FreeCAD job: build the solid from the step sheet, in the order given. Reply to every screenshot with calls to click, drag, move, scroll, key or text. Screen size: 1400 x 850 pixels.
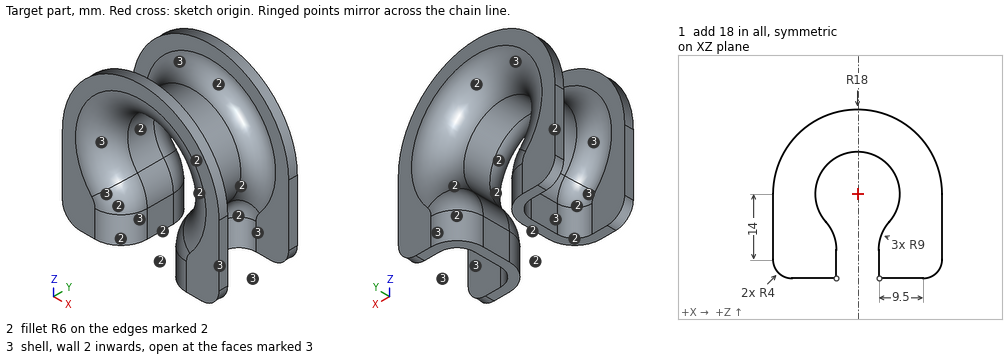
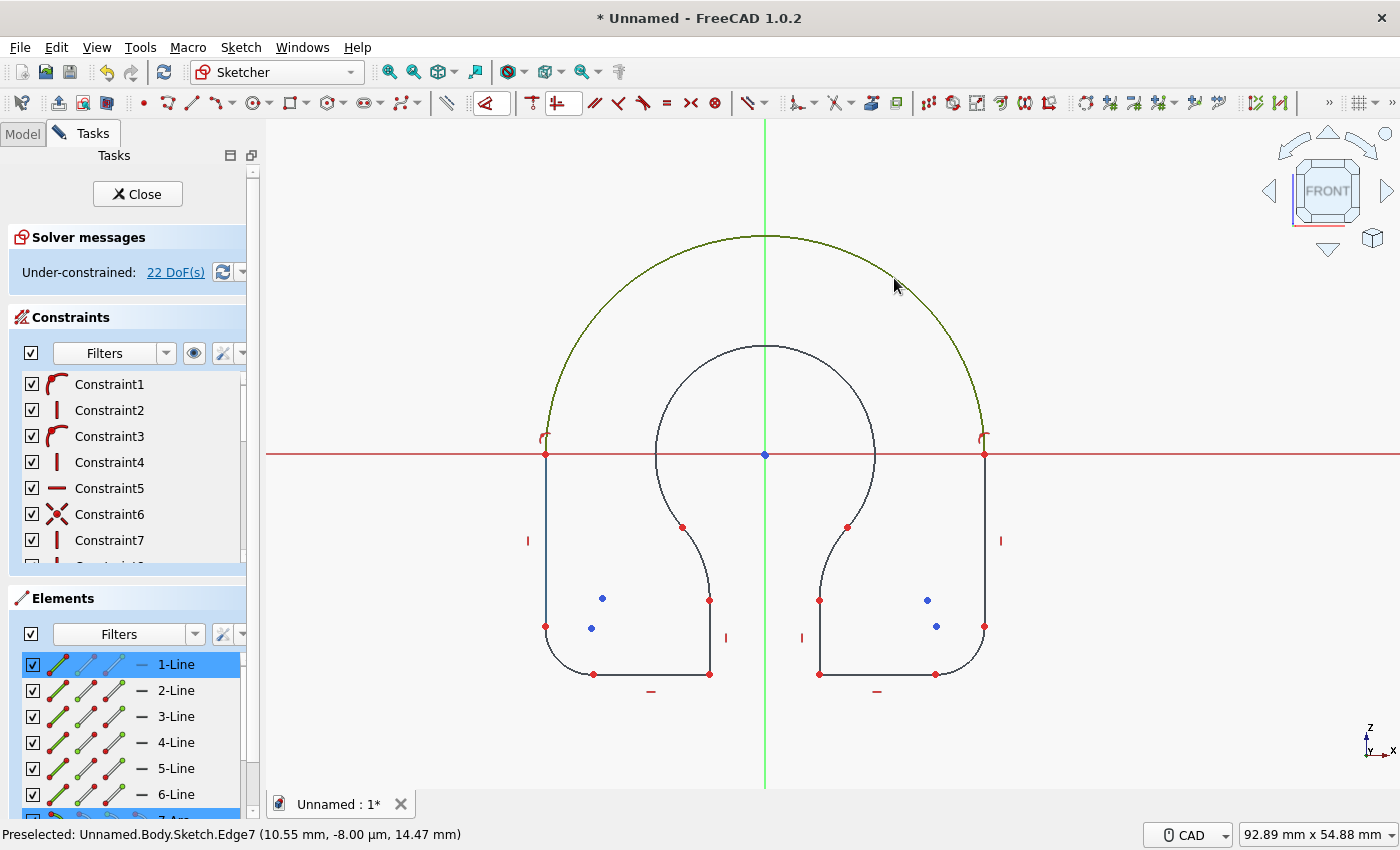
key(t)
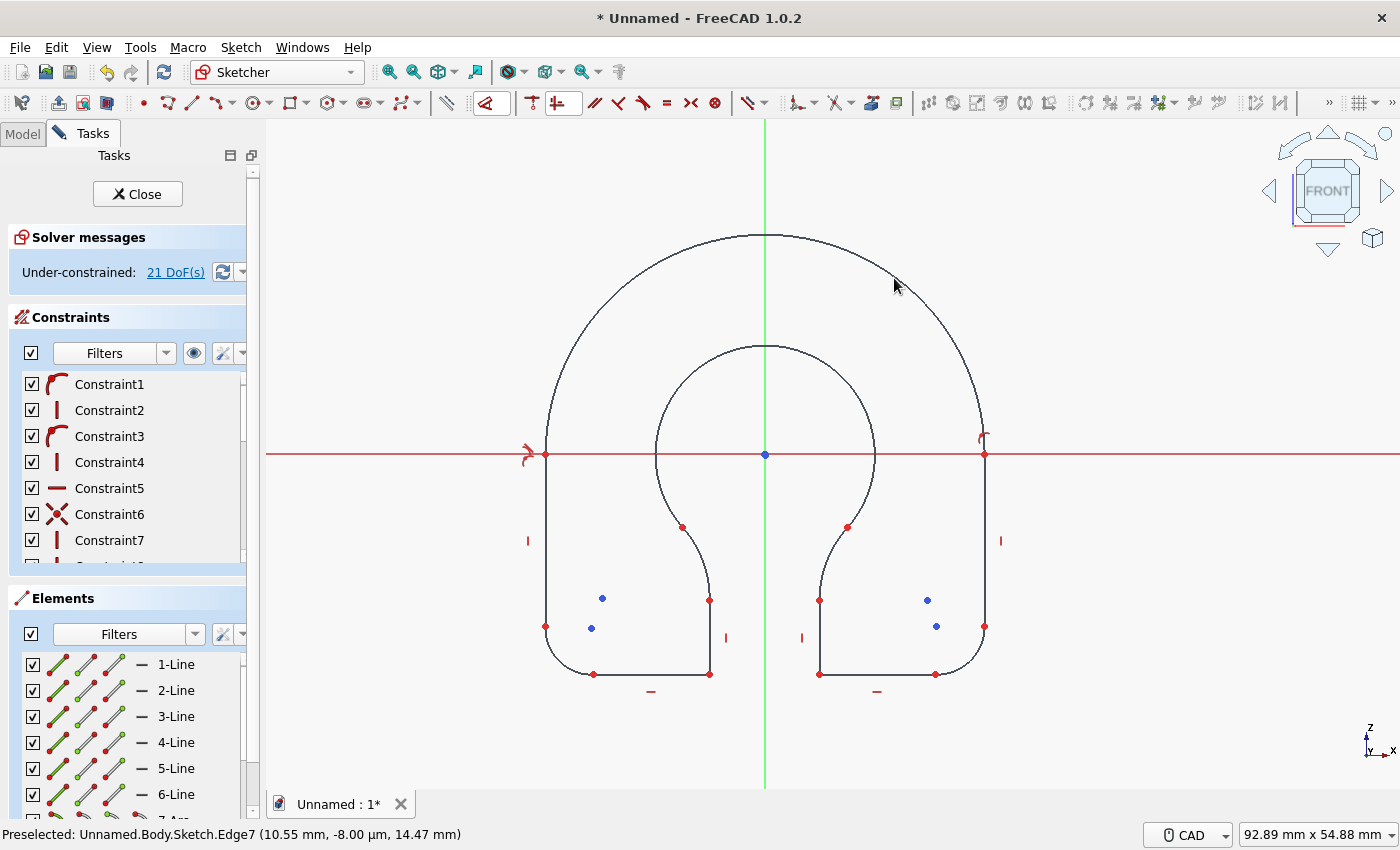
click(546, 575)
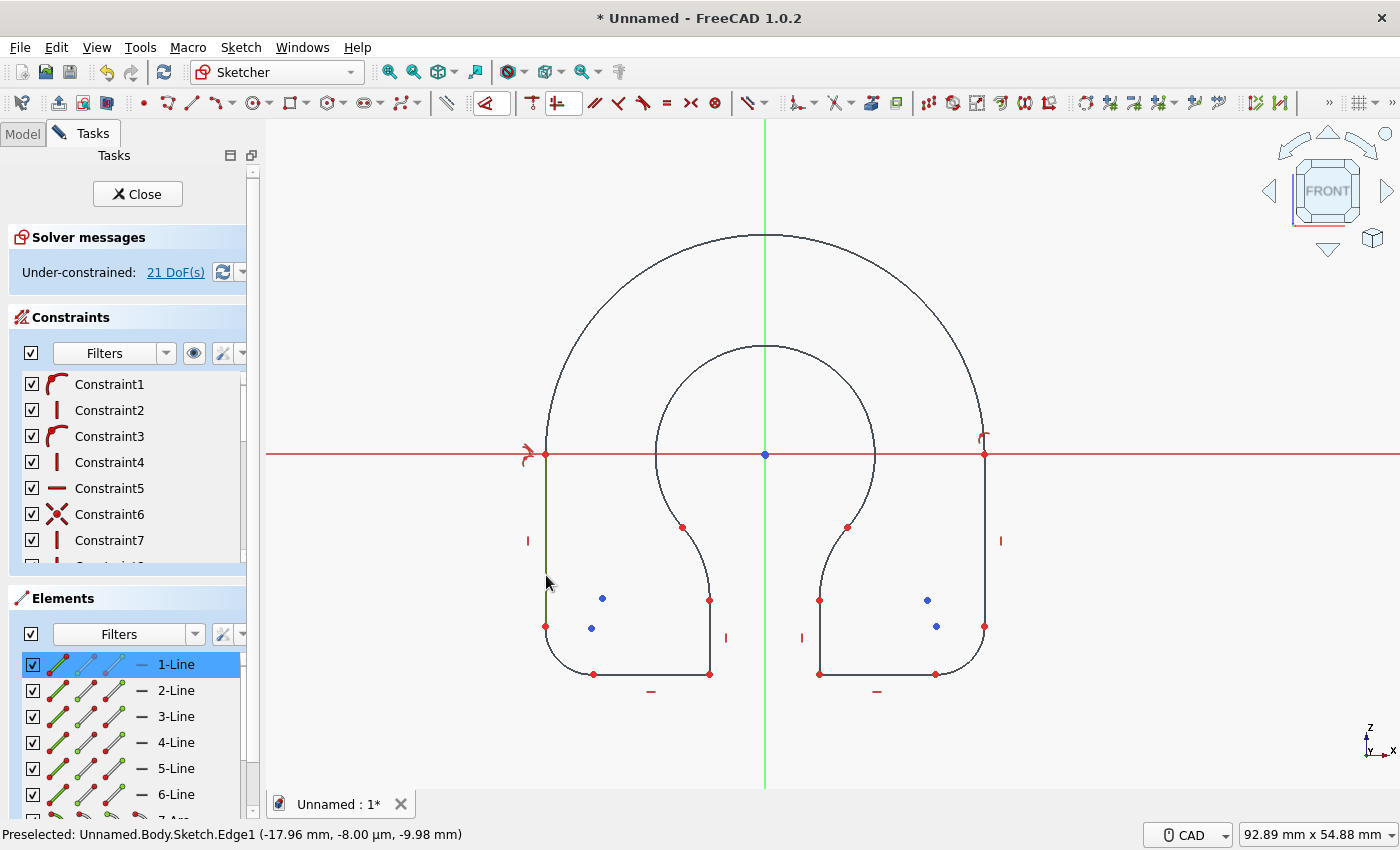
click(550, 649)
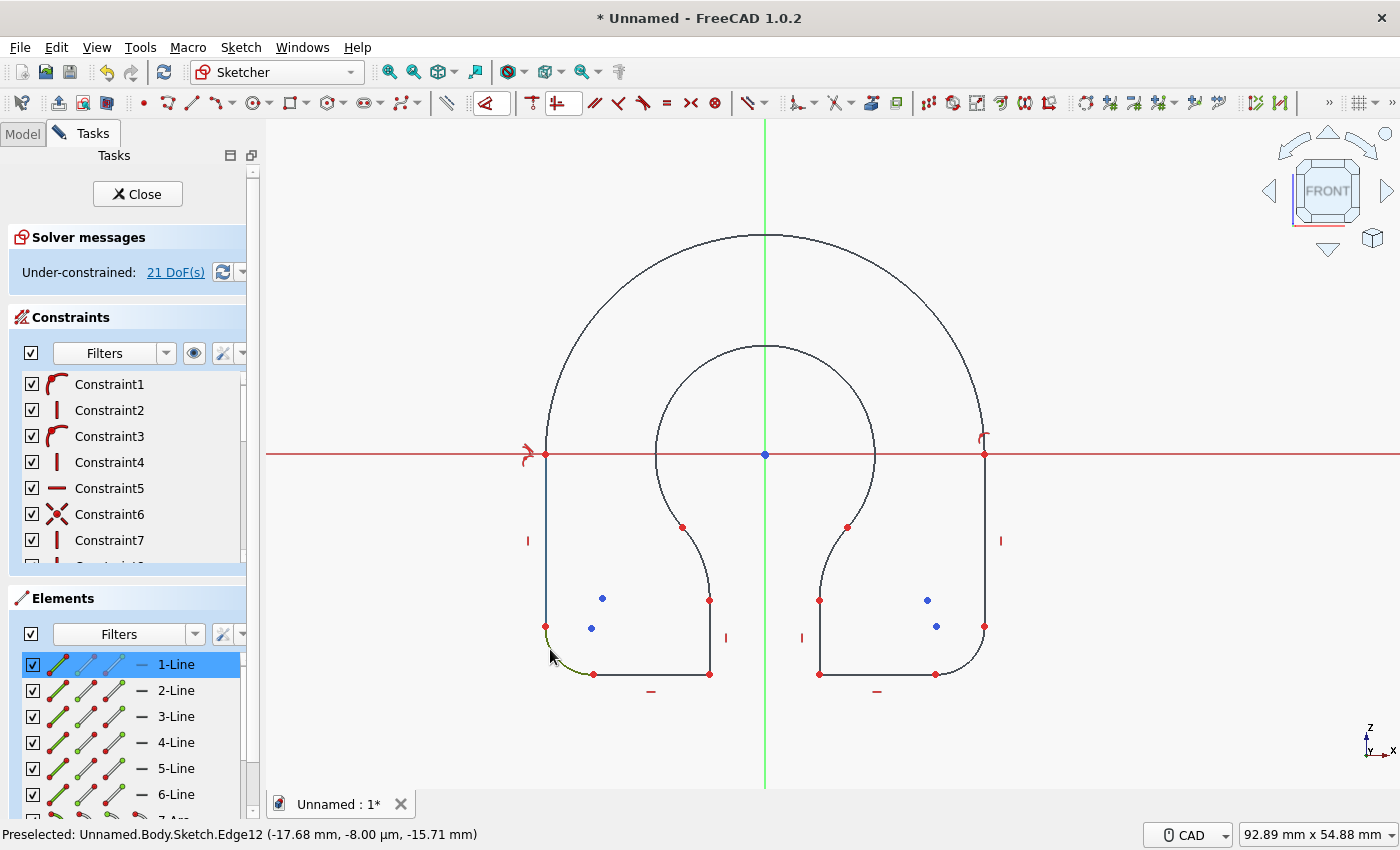
key(t)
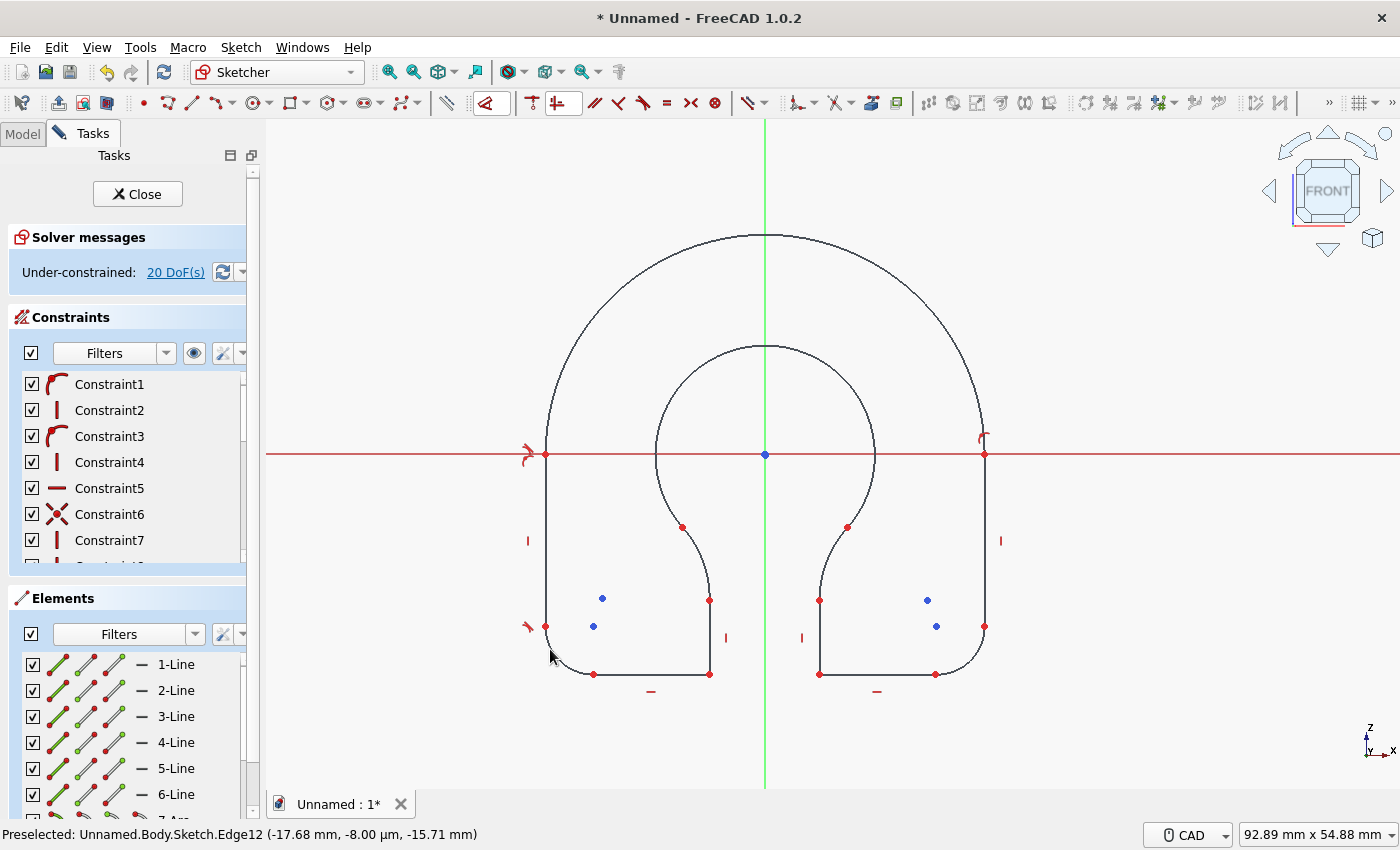
click(985, 506)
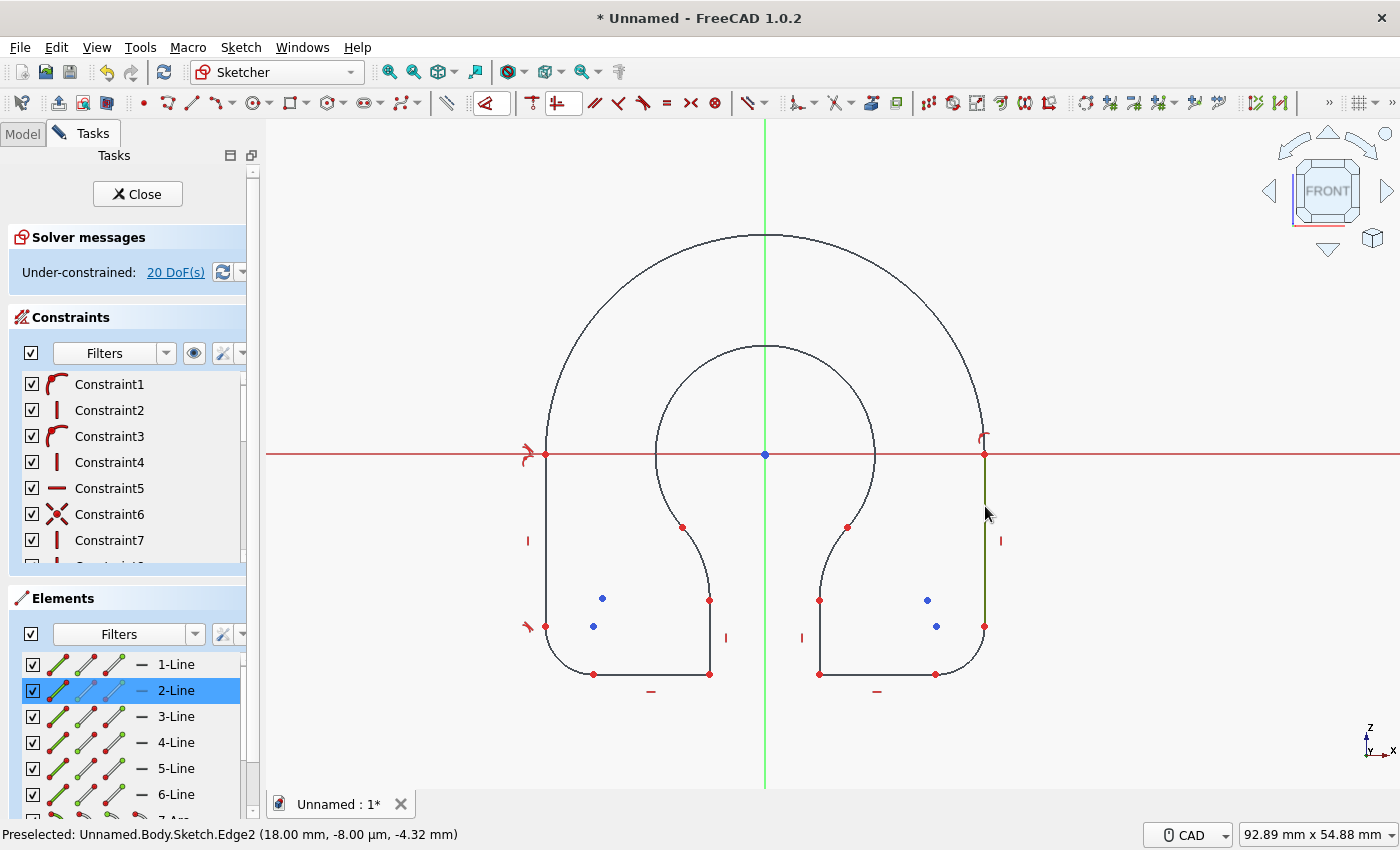
click(958, 670)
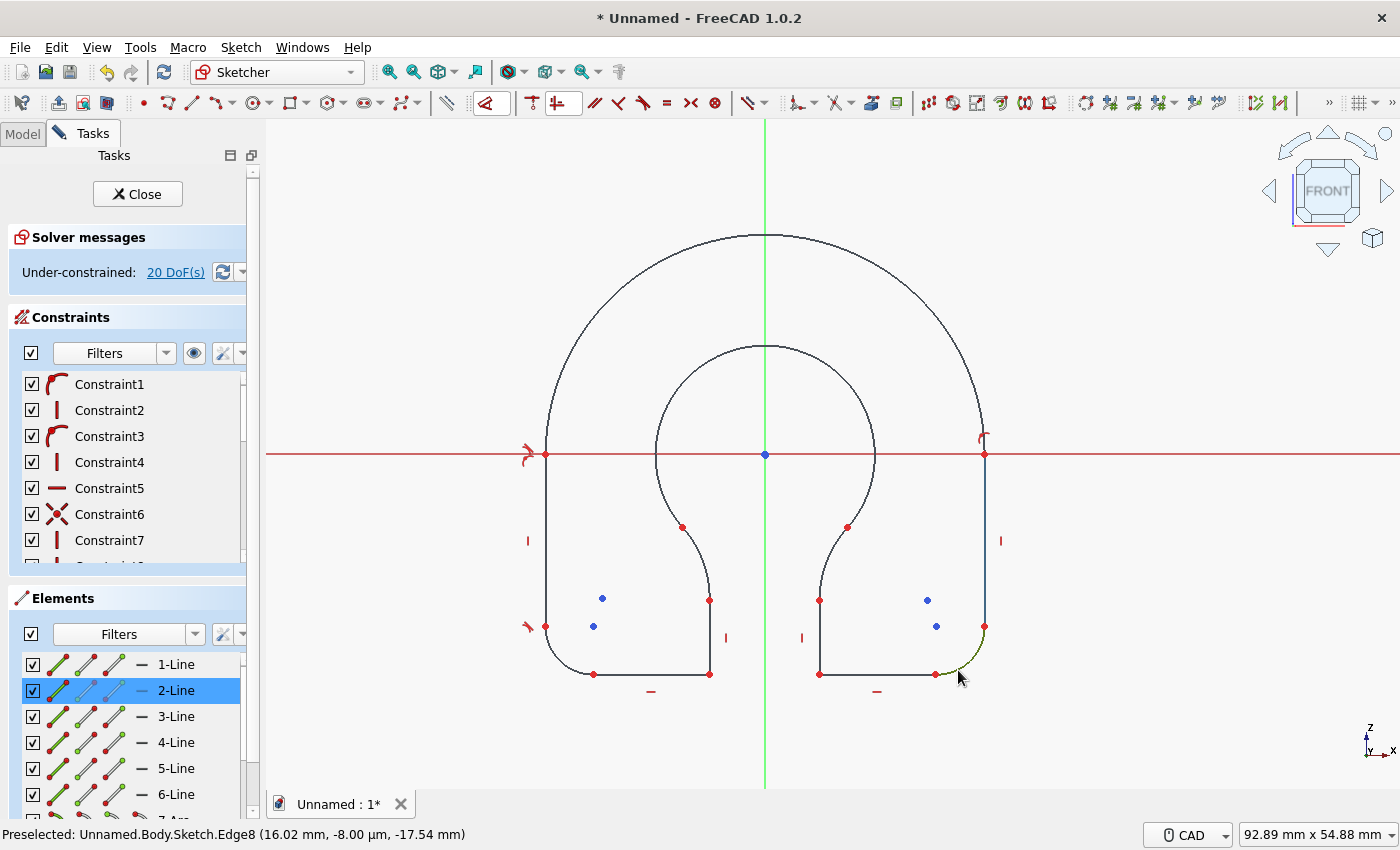
click(644, 104)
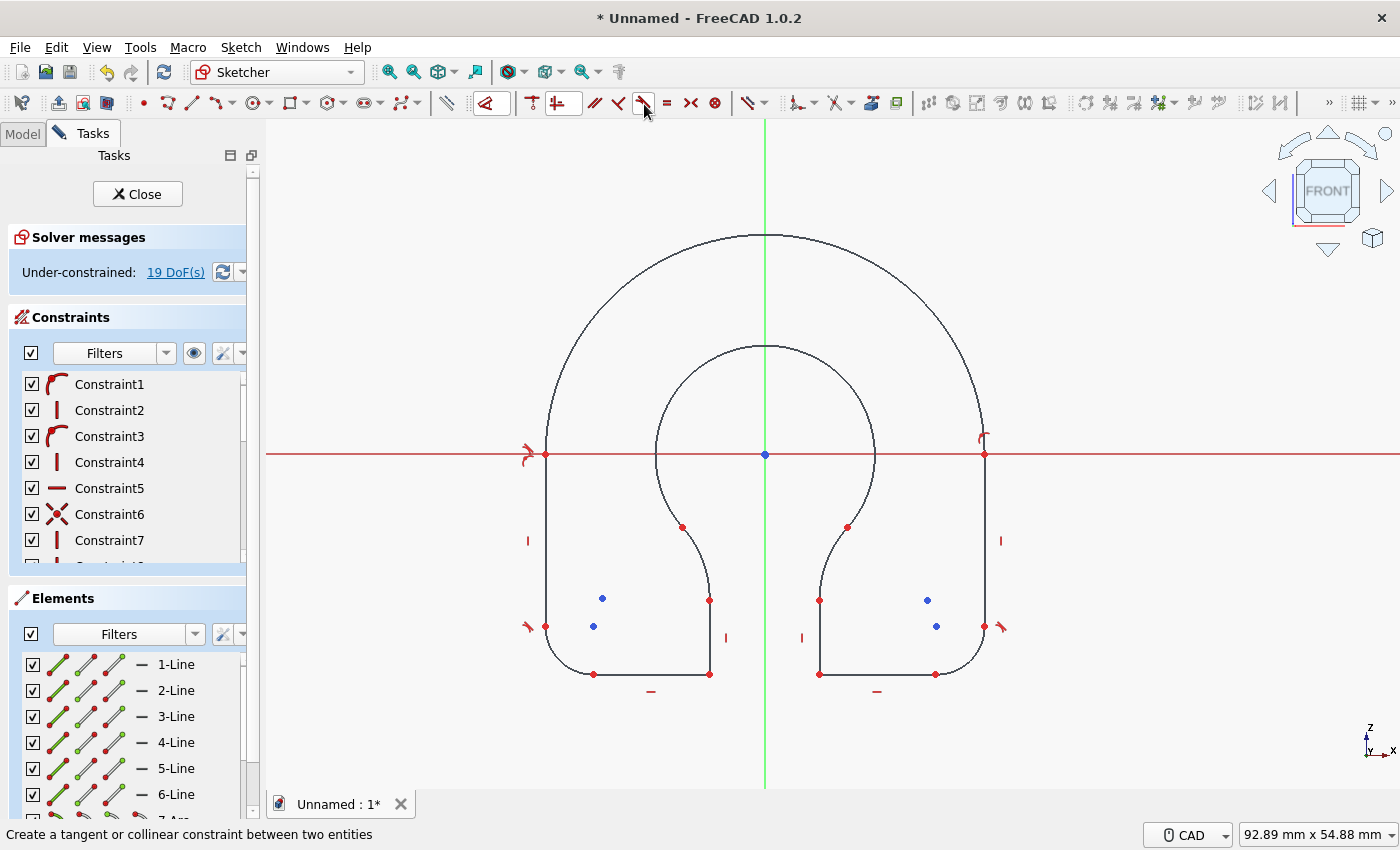
click(901, 675)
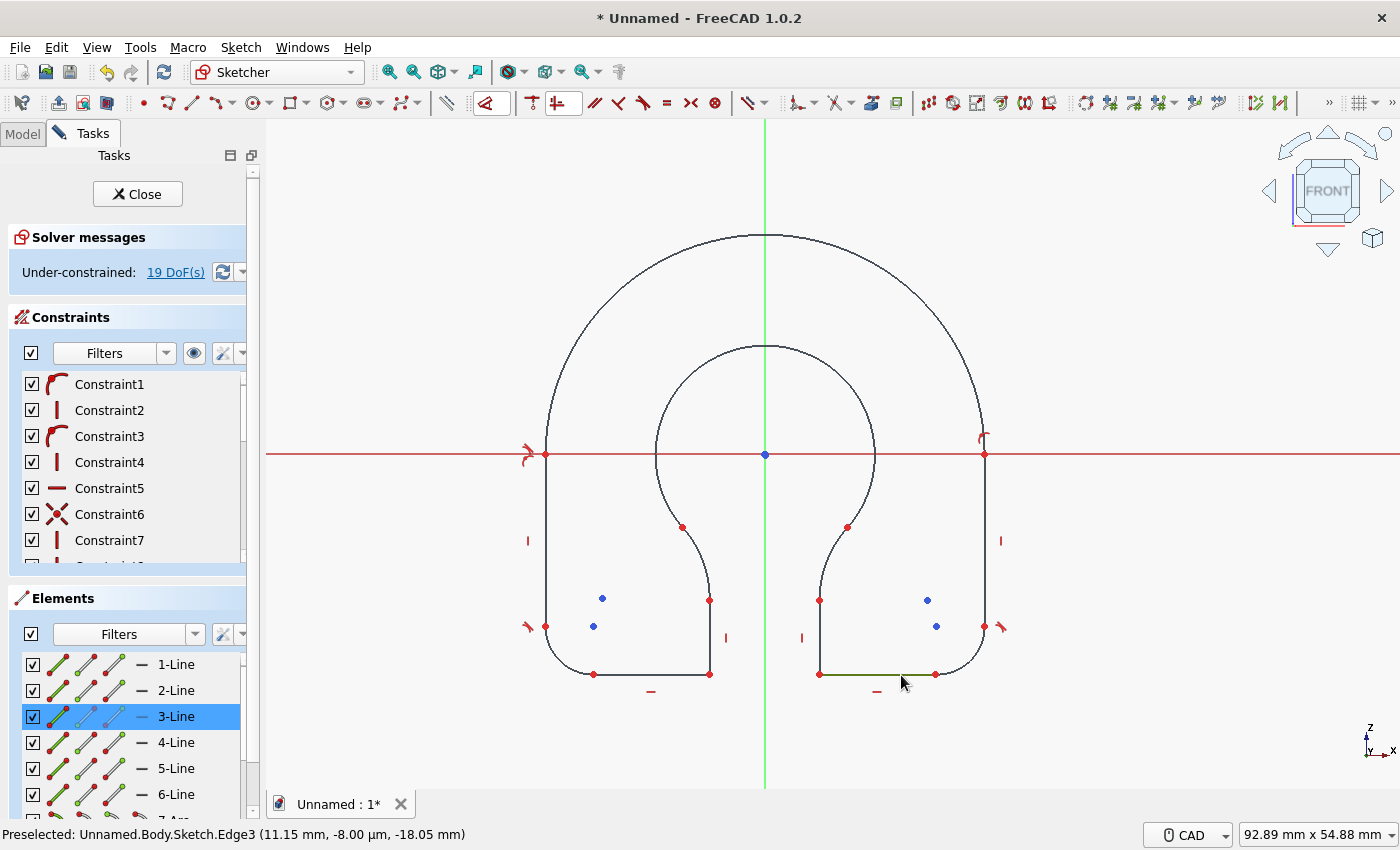
click(958, 670)